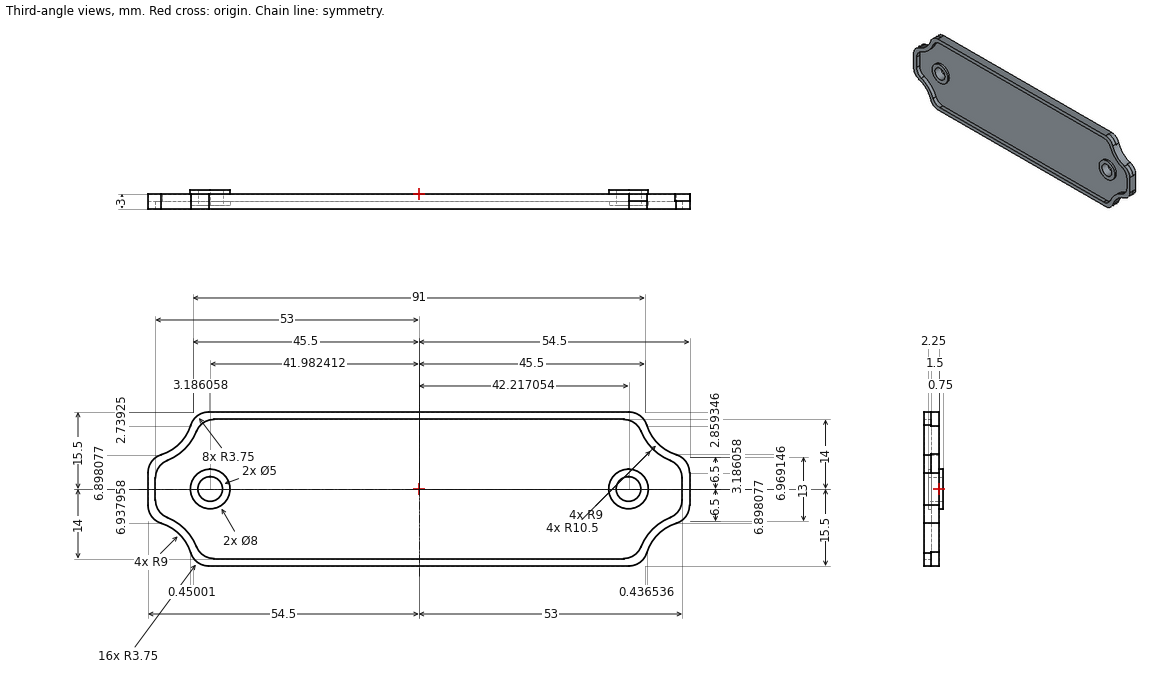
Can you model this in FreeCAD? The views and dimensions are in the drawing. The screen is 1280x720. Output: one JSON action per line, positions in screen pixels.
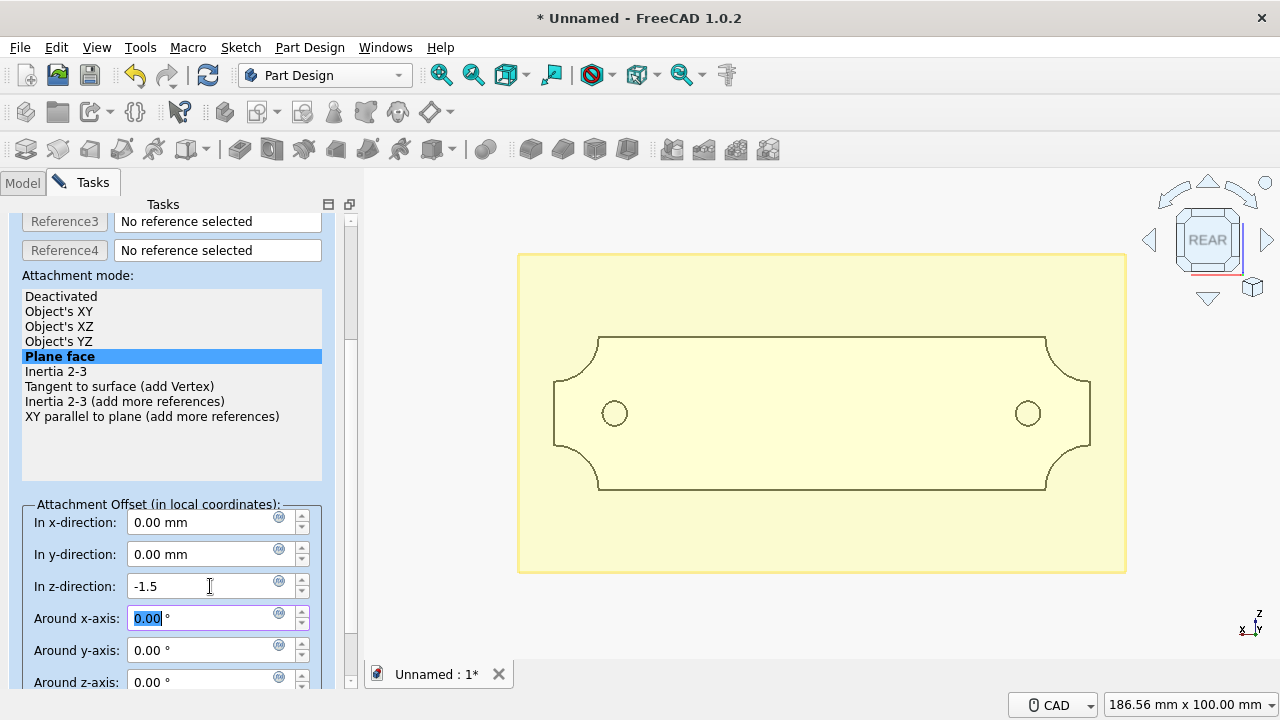
{"action": "scroll", "coordinate": [351, 451], "scroll_direction": "up", "scroll_amount": 4}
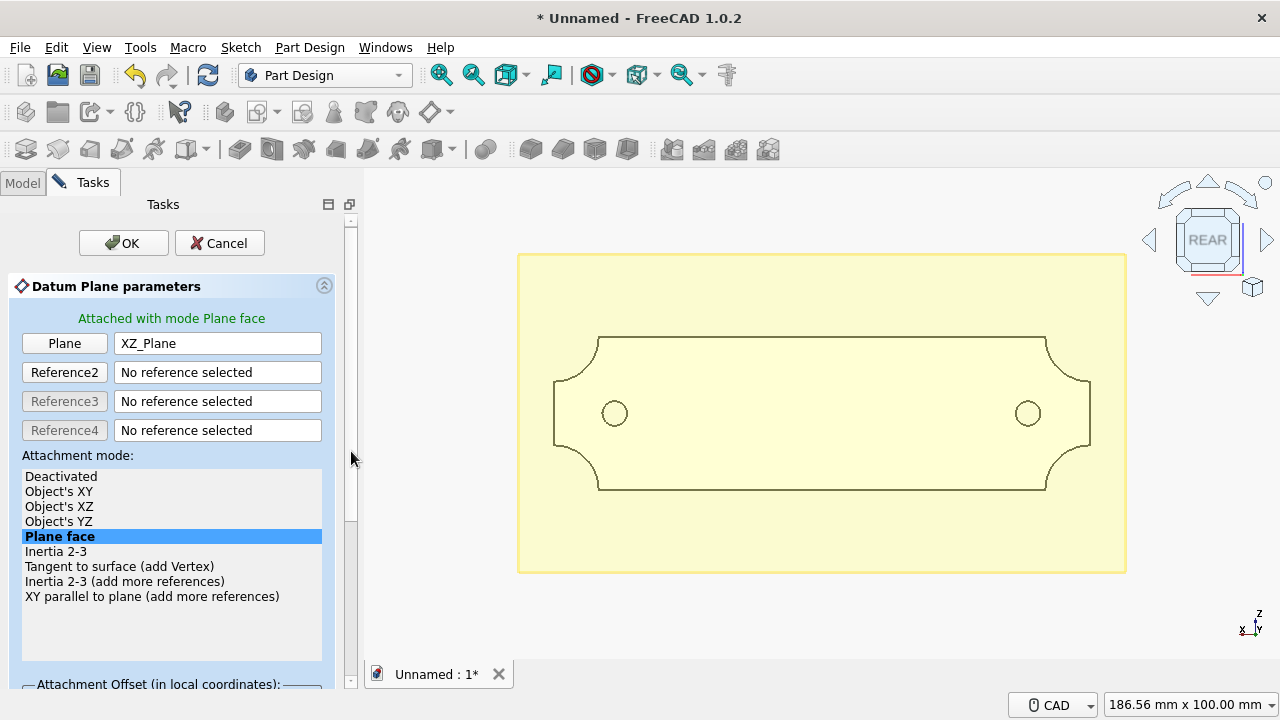
{"action": "left_click", "coordinate": [124, 243]}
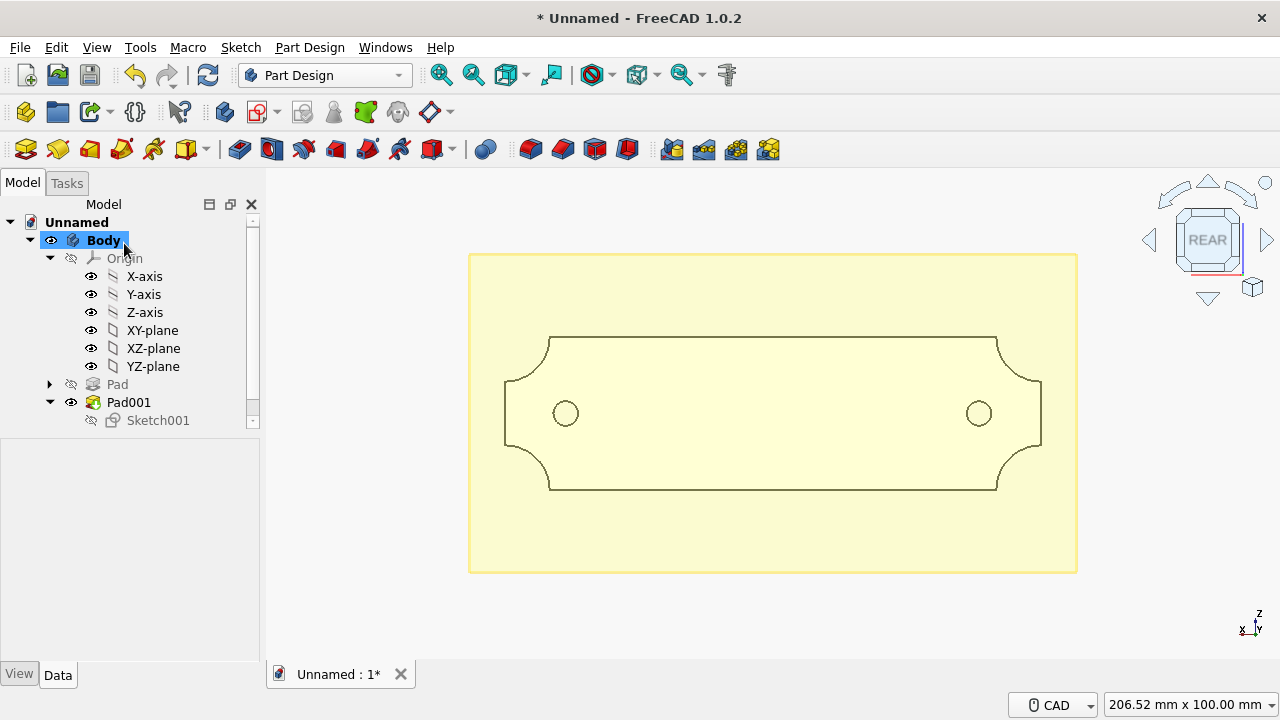
{"action": "scroll", "coordinate": [100, 326], "scroll_direction": "down", "scroll_amount": 3}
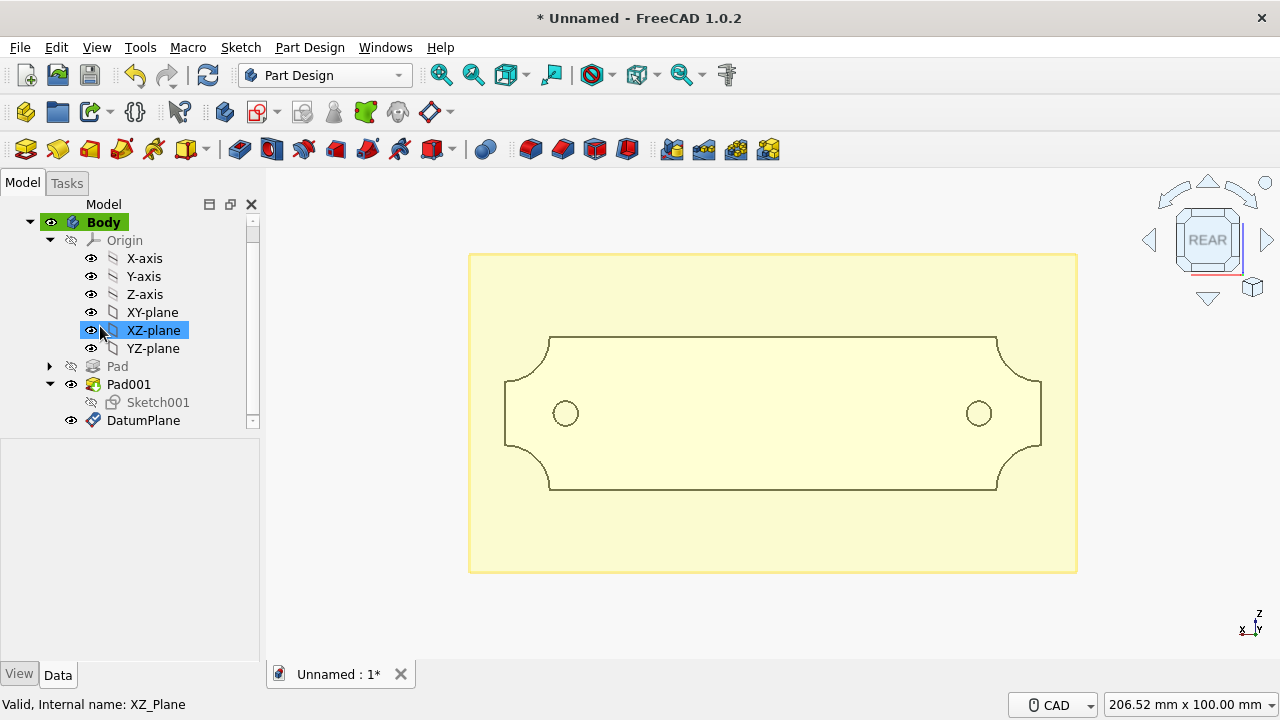
{"action": "left_click", "coordinate": [116, 420]}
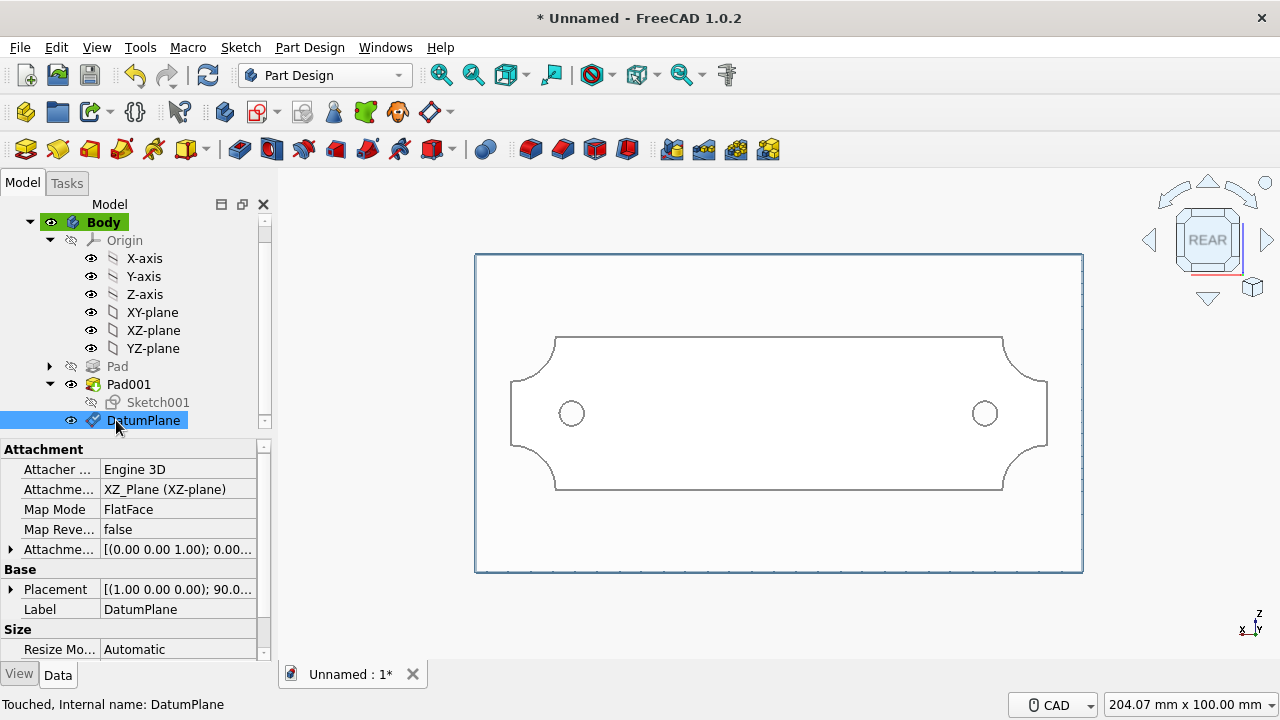
{"action": "left_click", "coordinate": [258, 112]}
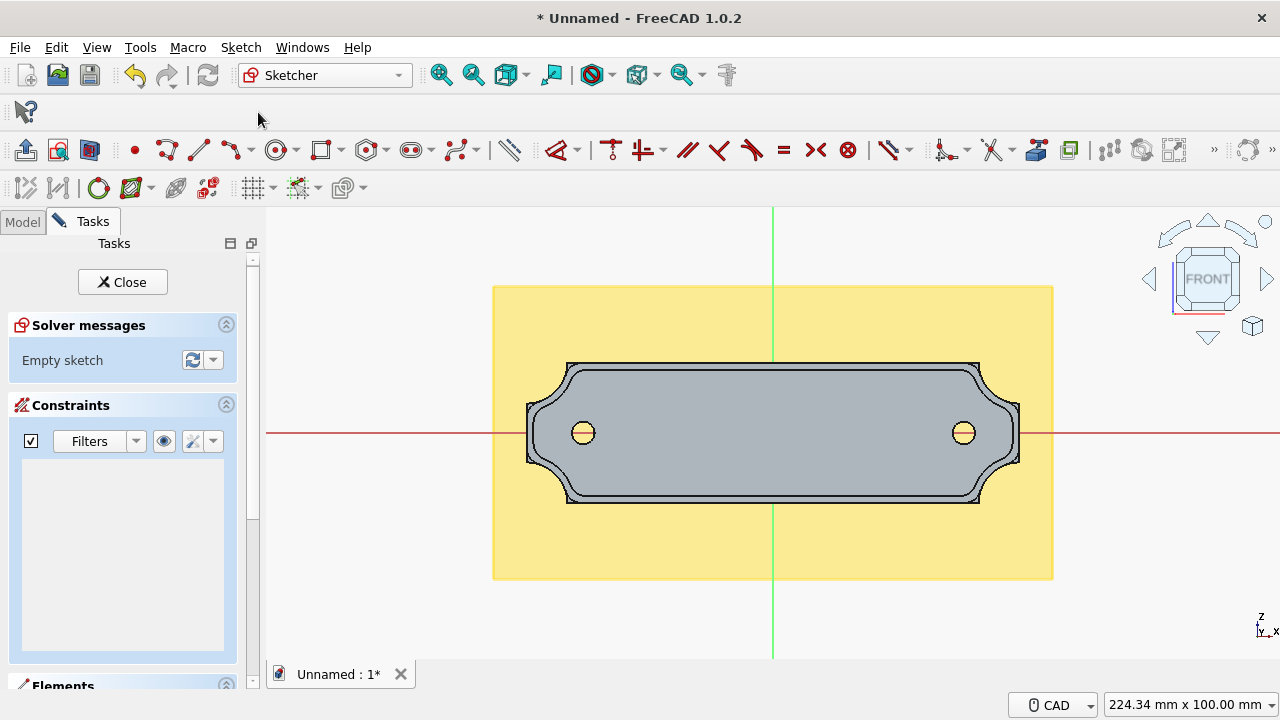
{"action": "left_click", "coordinate": [90, 150]}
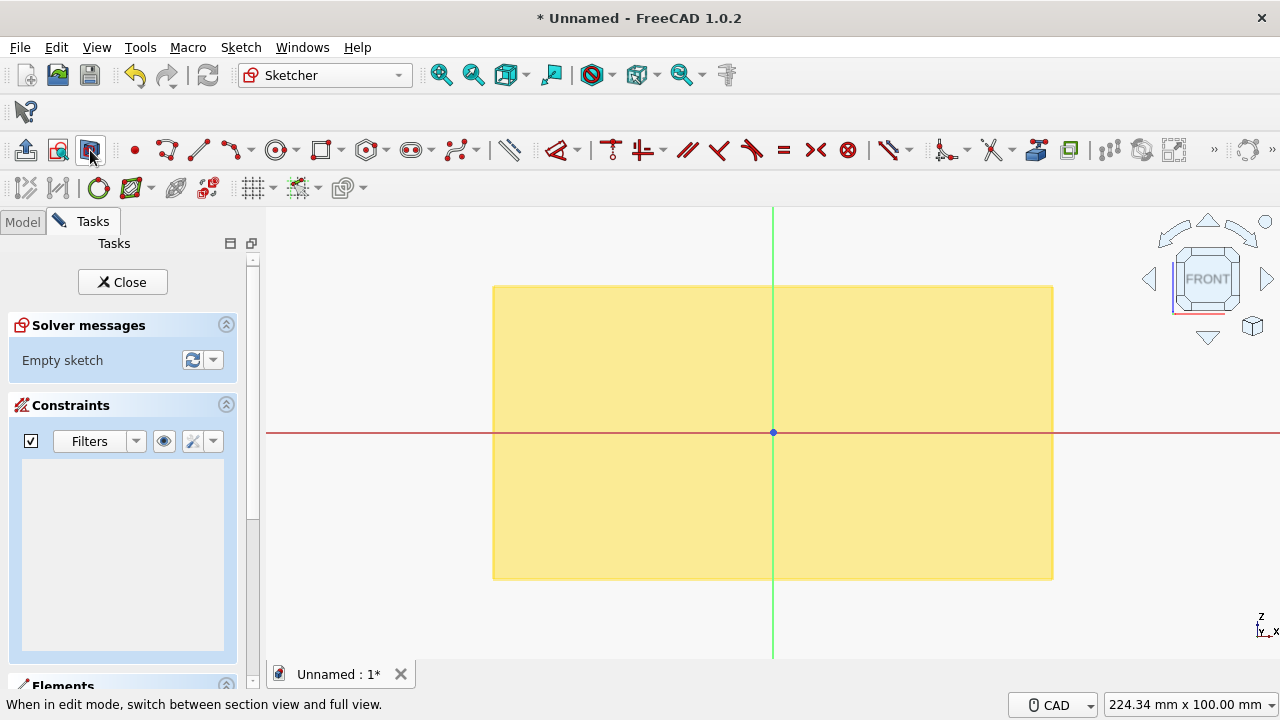
{"action": "left_click", "coordinate": [168, 150]}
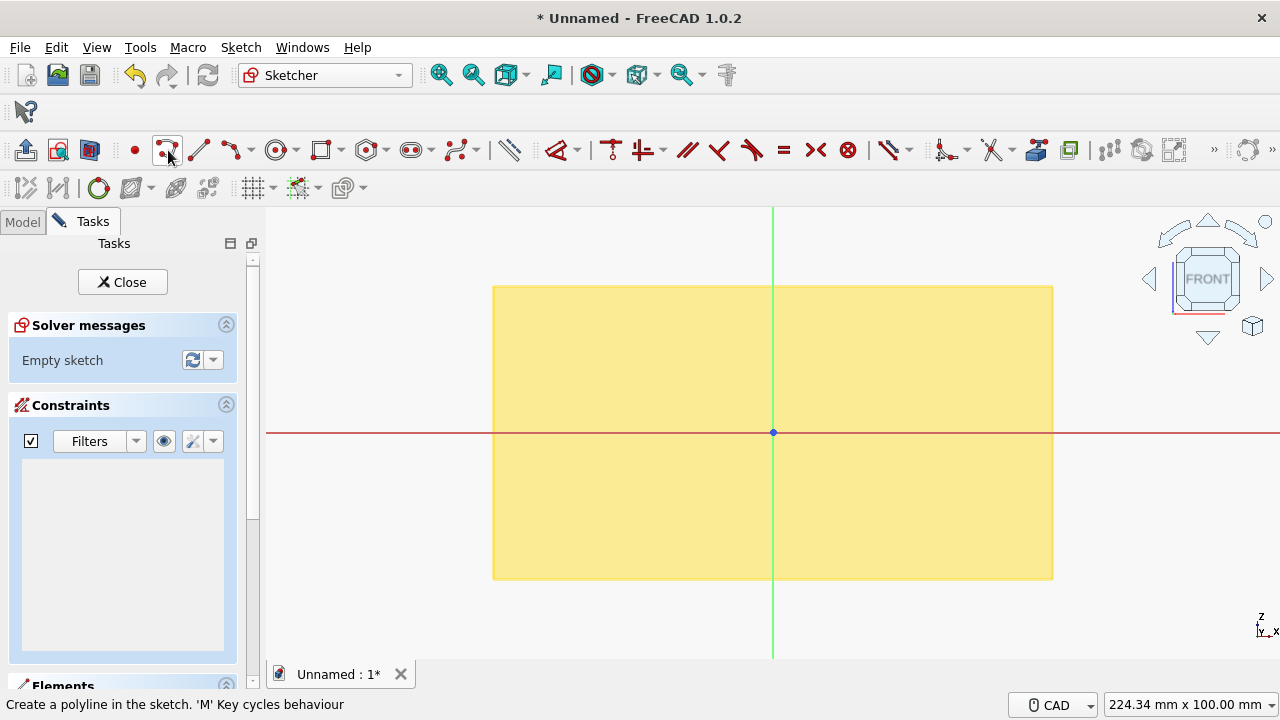
{"action": "left_click", "coordinate": [582, 363]}
{"action": "left_click", "coordinate": [567, 363]}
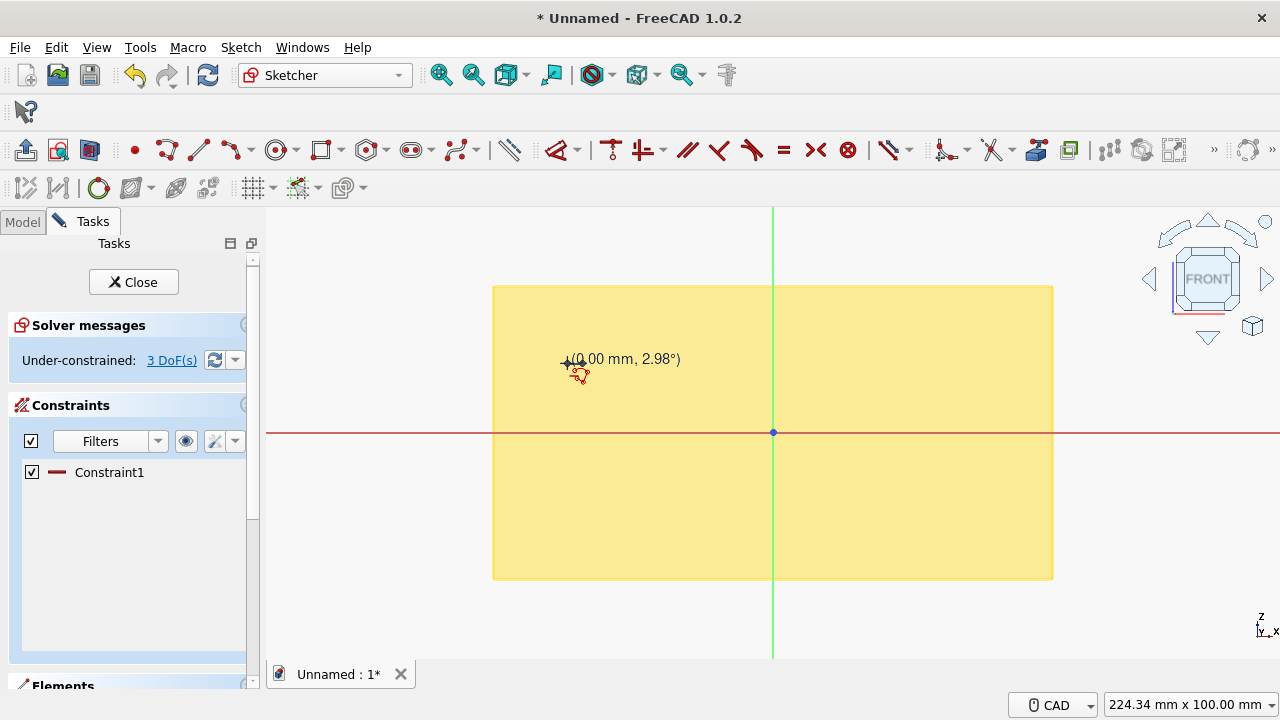
{"action": "scroll", "coordinate": [565, 375], "scroll_direction": "up", "scroll_amount": 2}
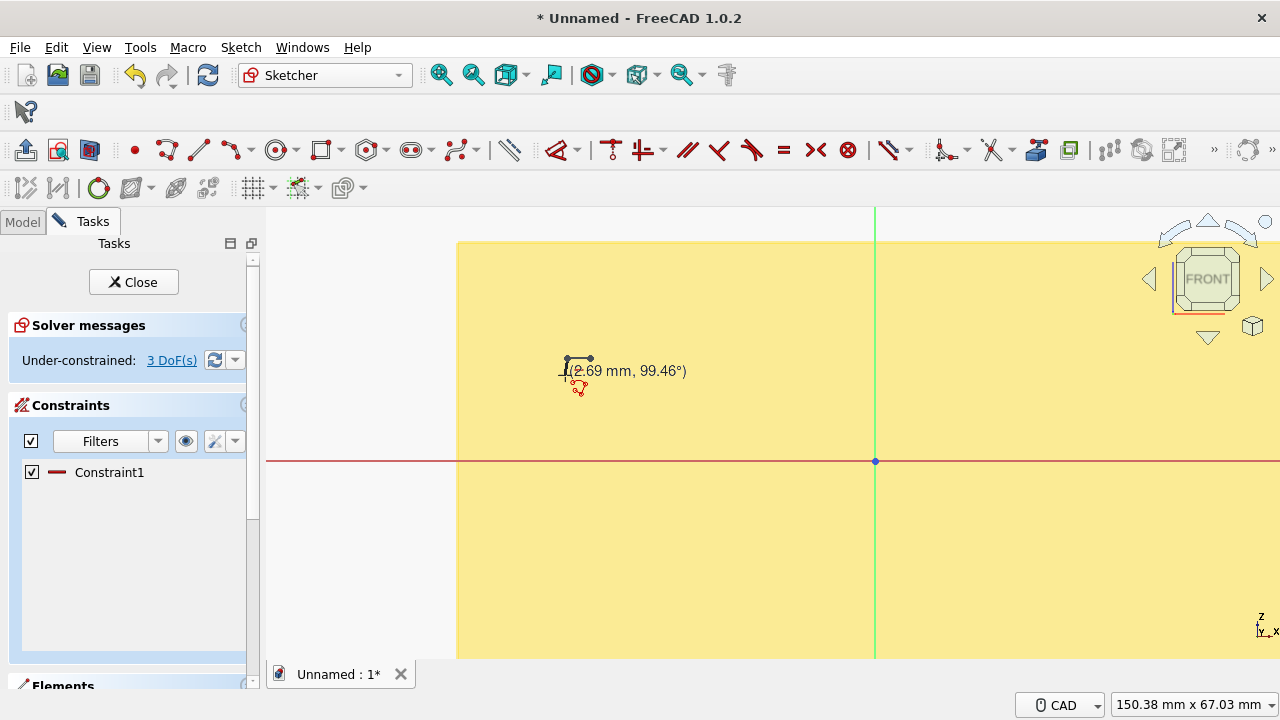
{"action": "left_click", "coordinate": [565, 375]}
{"action": "right_click", "coordinate": [565, 375]}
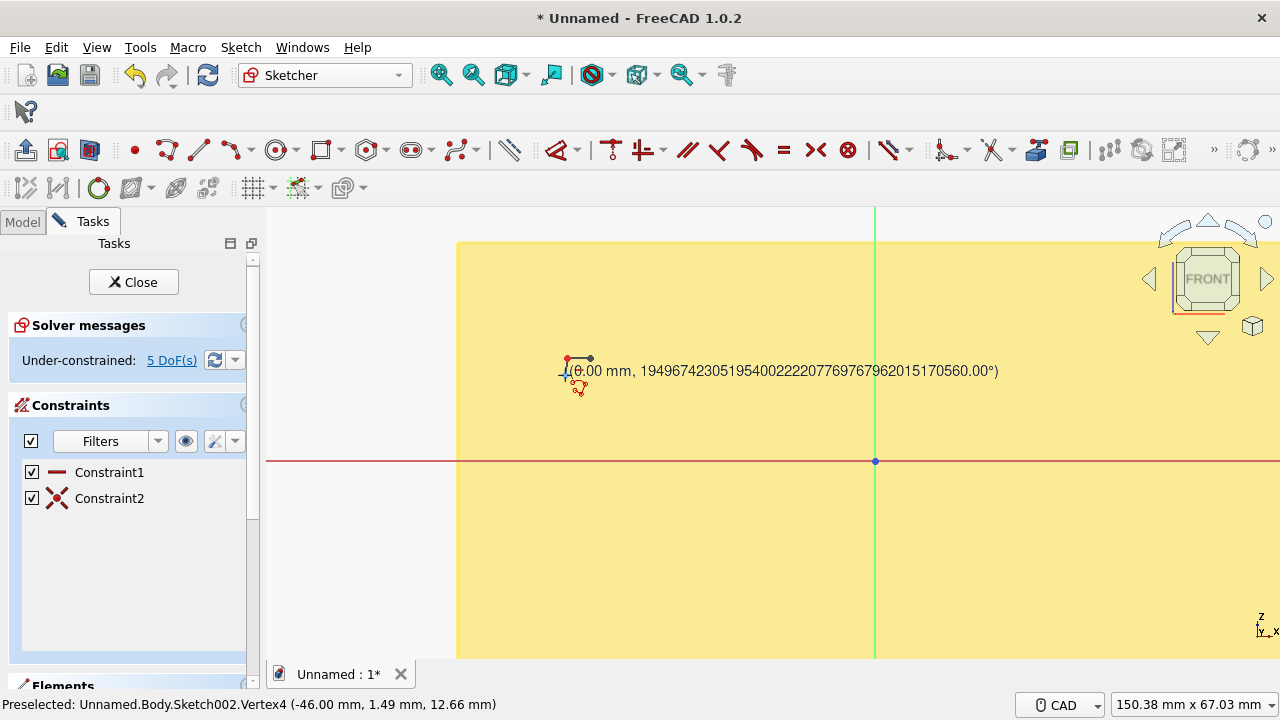
{"action": "left_click", "coordinate": [232, 150]}